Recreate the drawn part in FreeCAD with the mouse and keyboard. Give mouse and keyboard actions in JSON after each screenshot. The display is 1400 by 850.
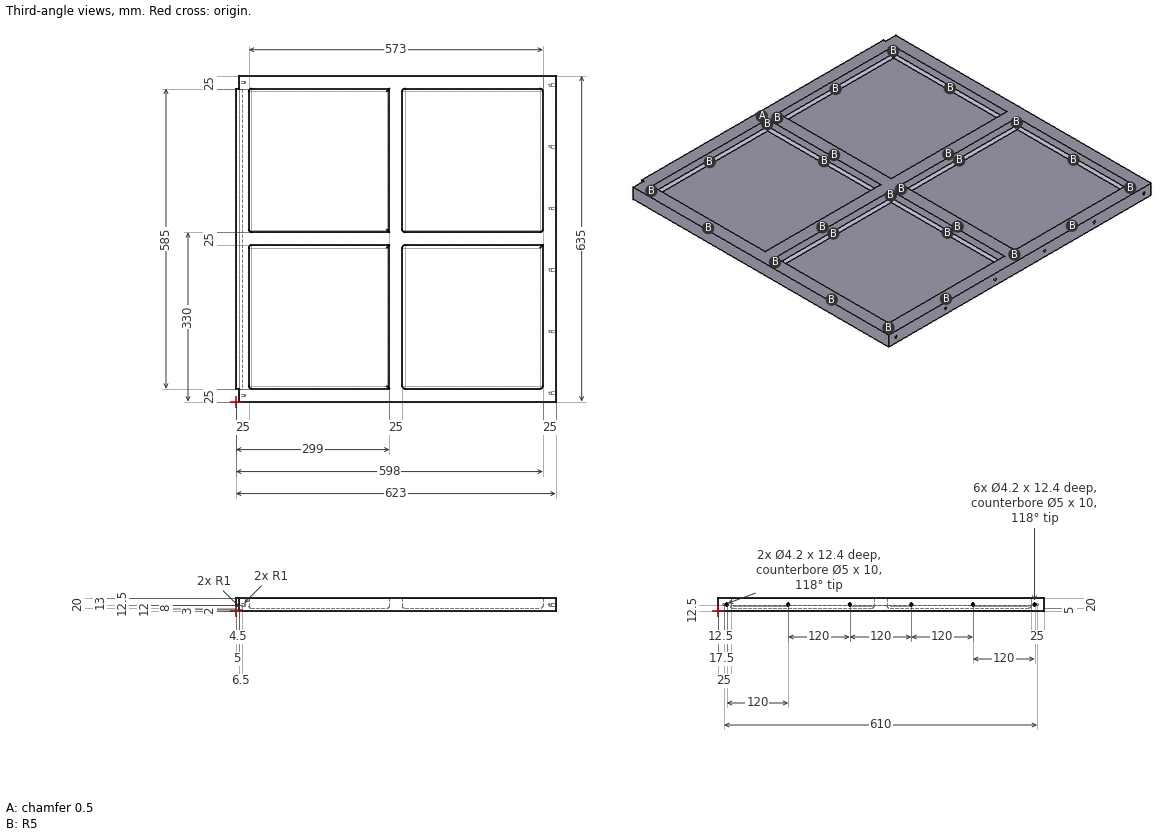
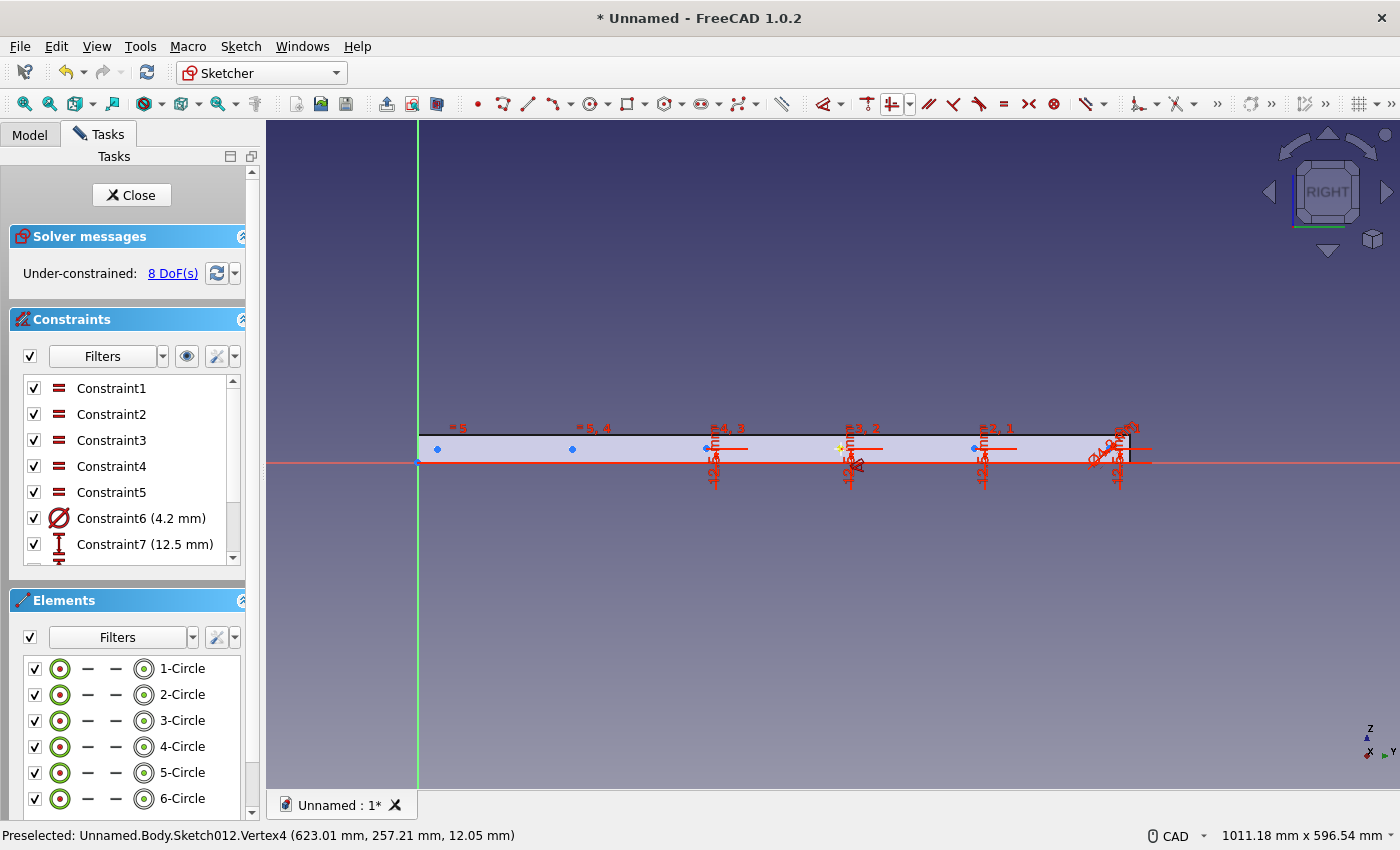
{"action": "scroll", "coordinate": [572, 449], "scroll_direction": "up", "scroll_amount": 6}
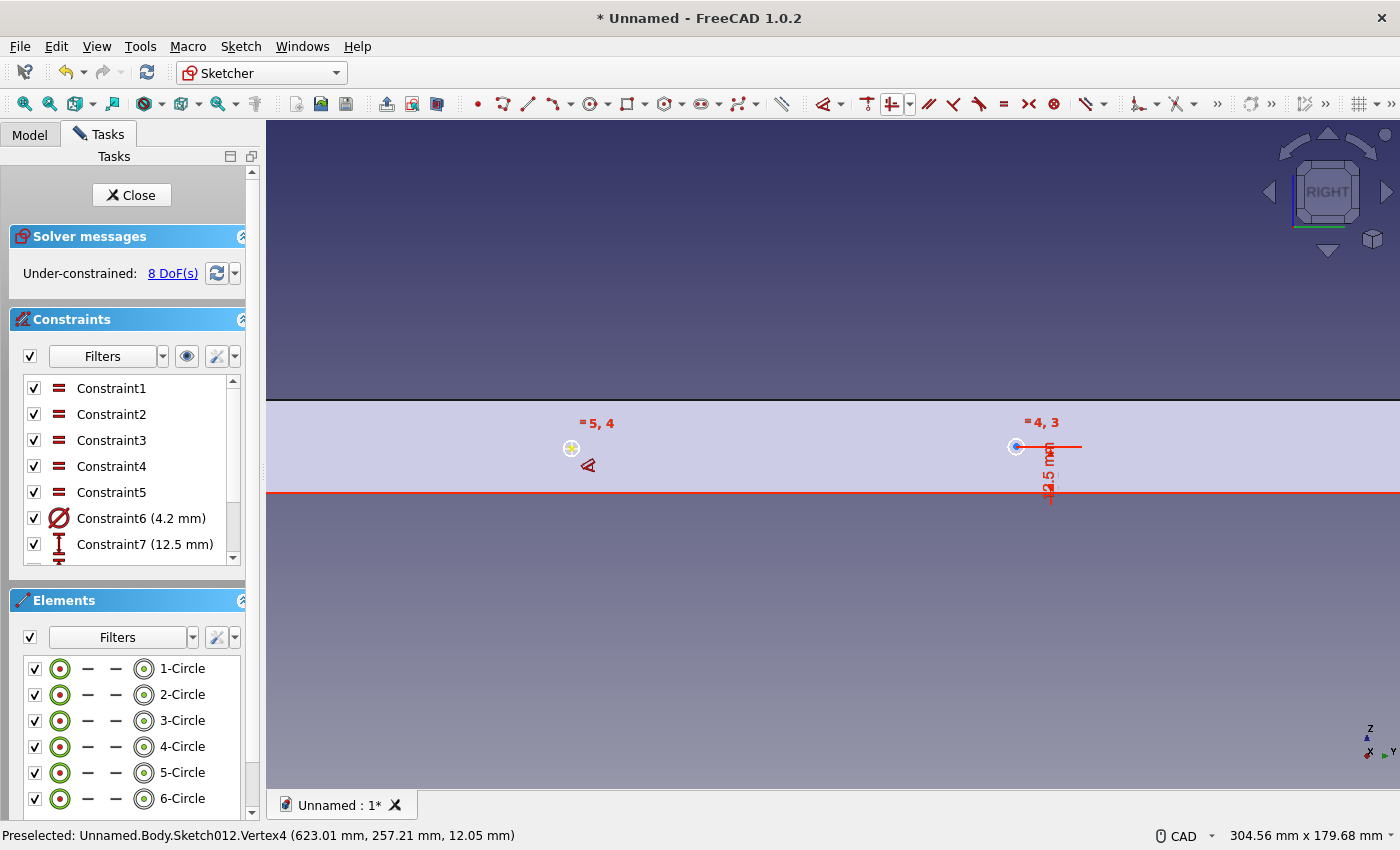
{"action": "left_click", "coordinate": [571, 448]}
{"action": "left_click", "coordinate": [605, 471]}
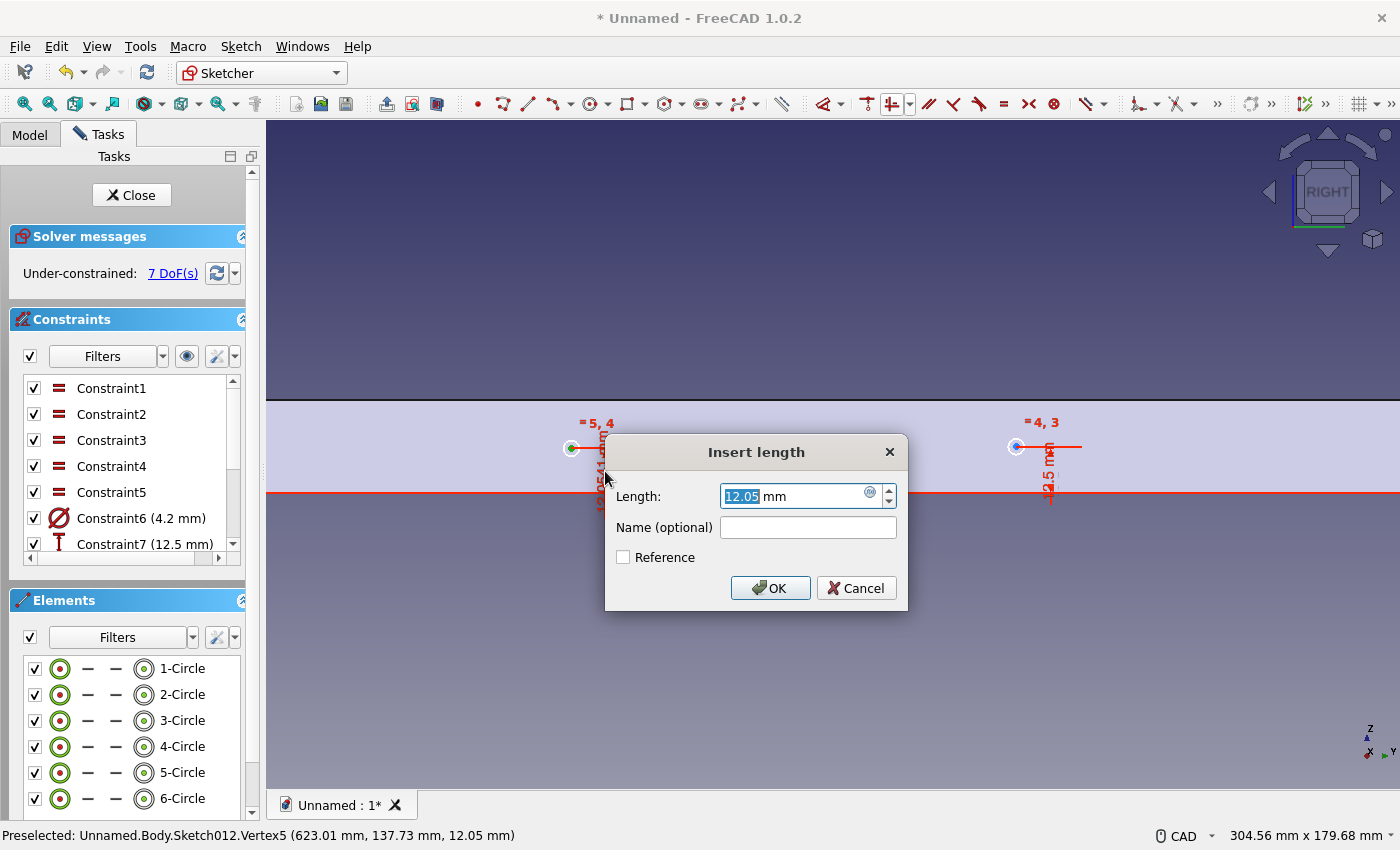
{"action": "type", "text": "12.5"}
{"action": "key", "text": "Return"}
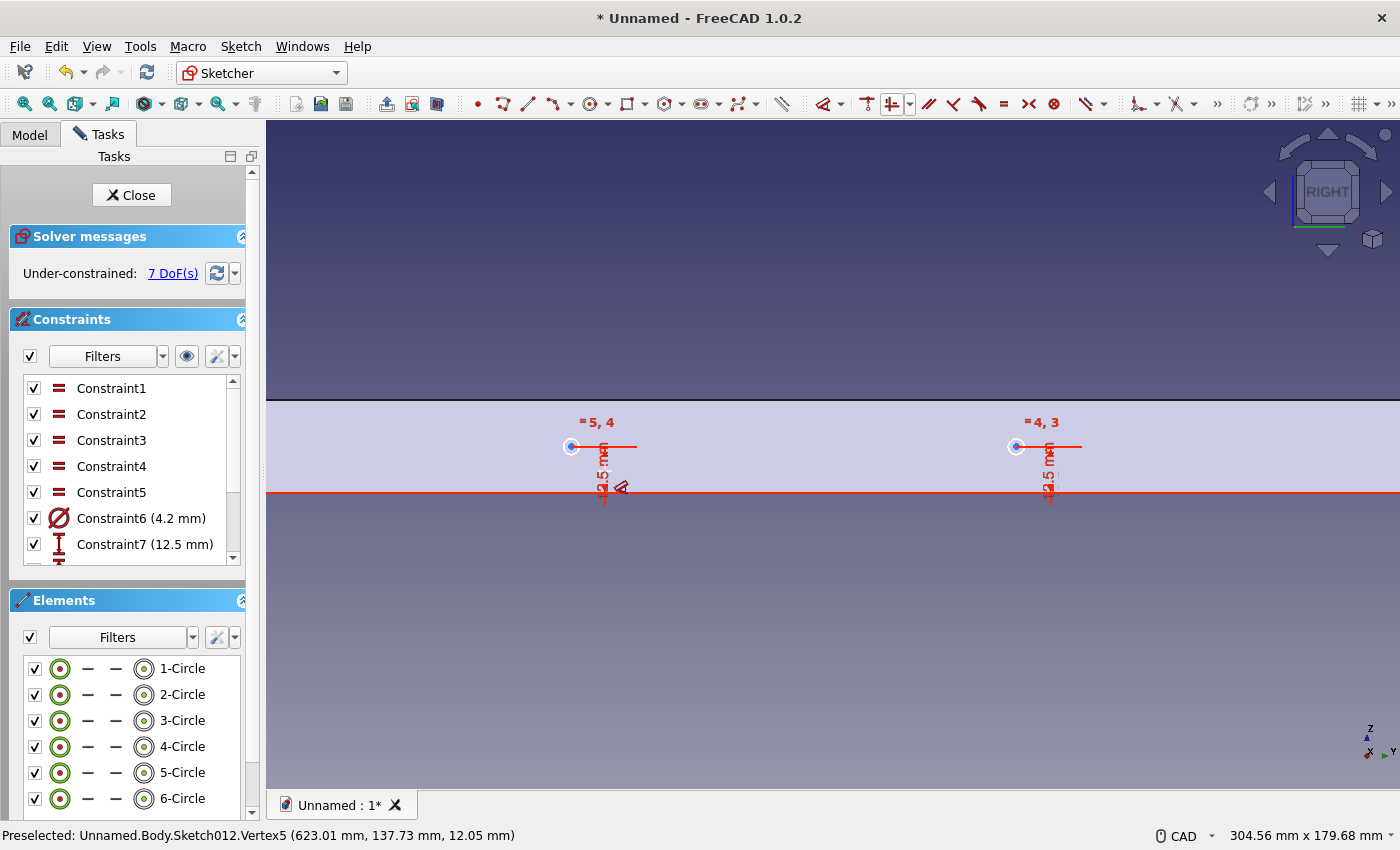
{"action": "scroll", "coordinate": [572, 449], "scroll_direction": "down", "scroll_amount": 6}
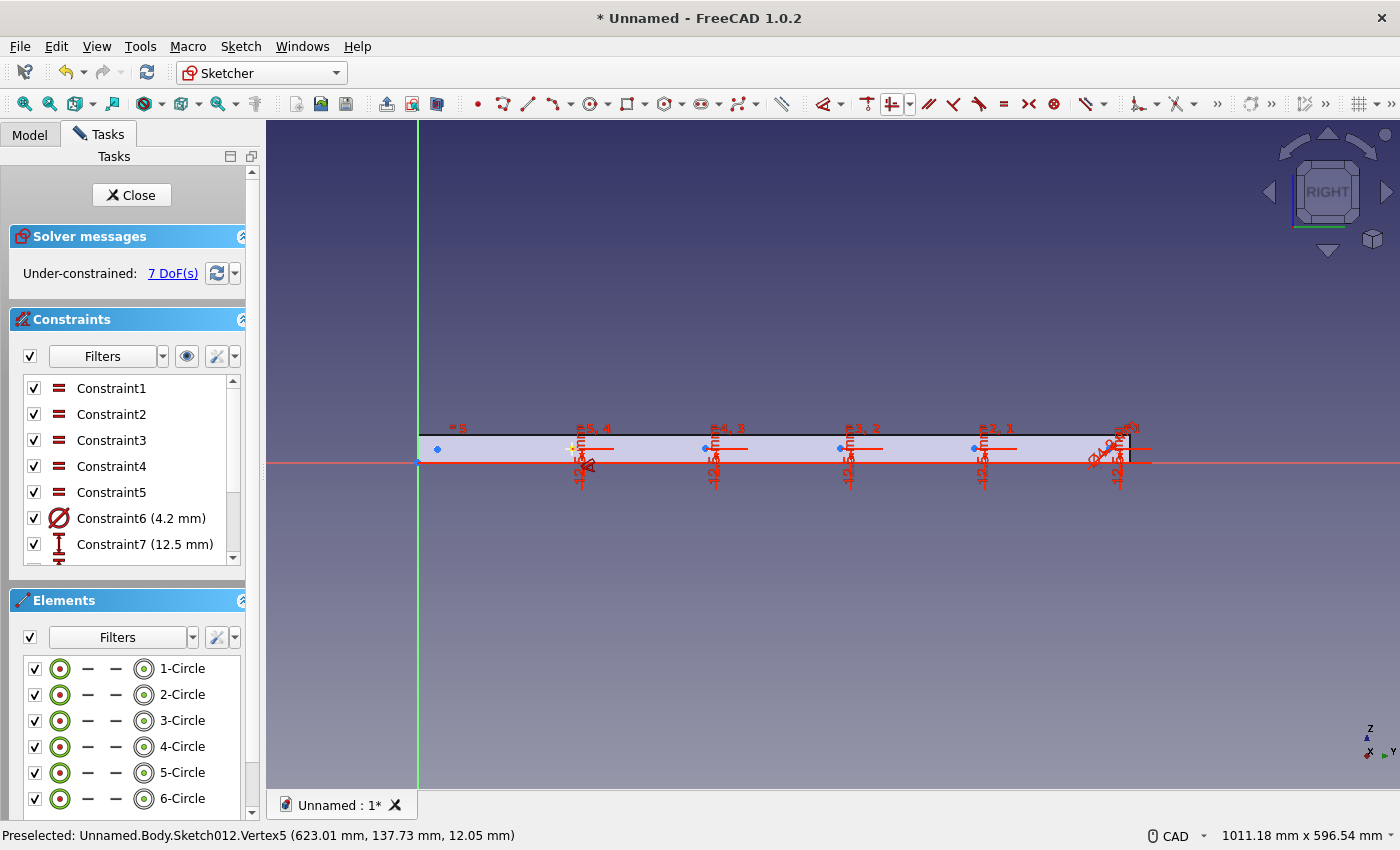
{"action": "scroll", "coordinate": [437, 449], "scroll_direction": "up", "scroll_amount": 4}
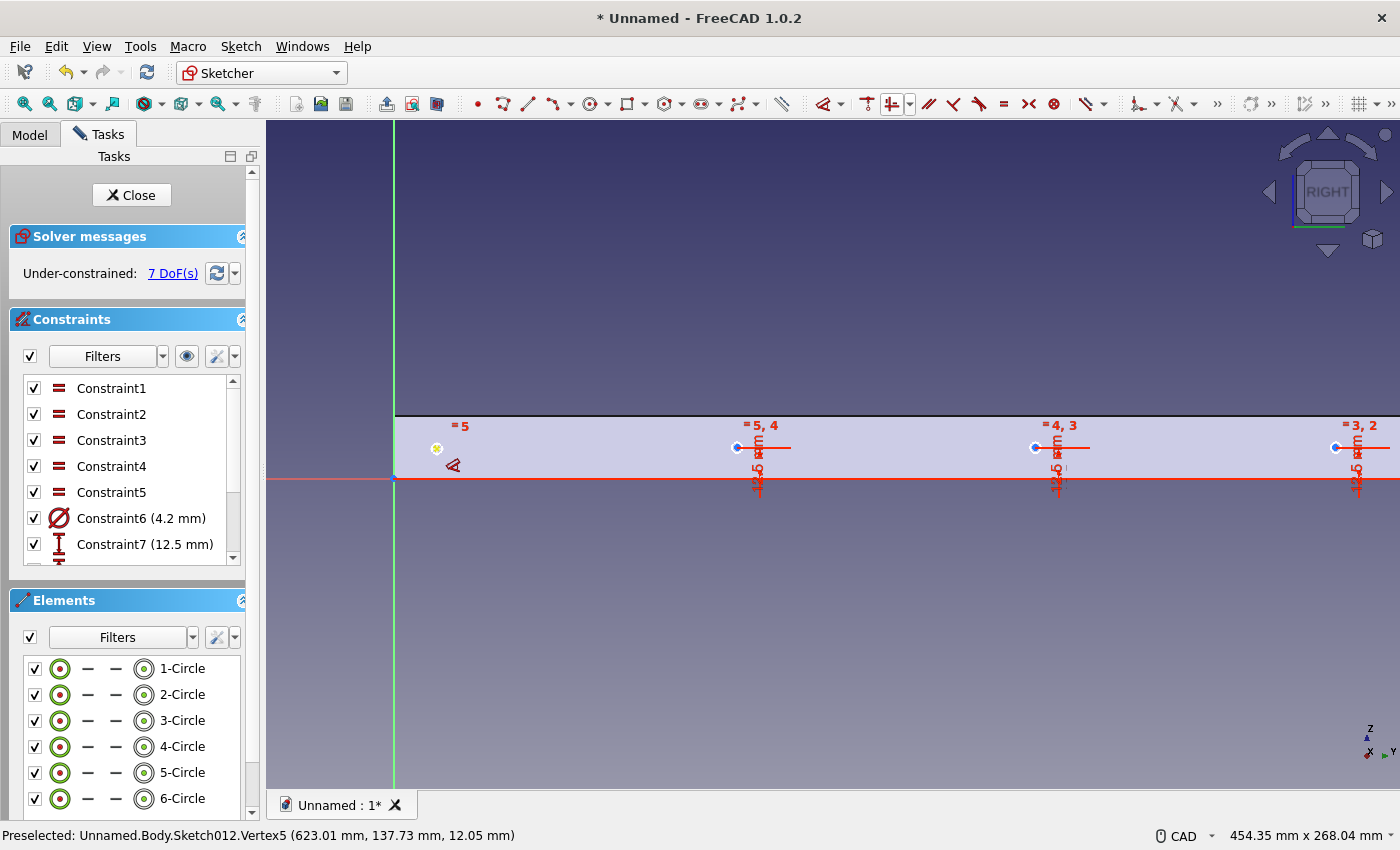
{"action": "left_click", "coordinate": [437, 449]}
{"action": "left_click", "coordinate": [415, 513]}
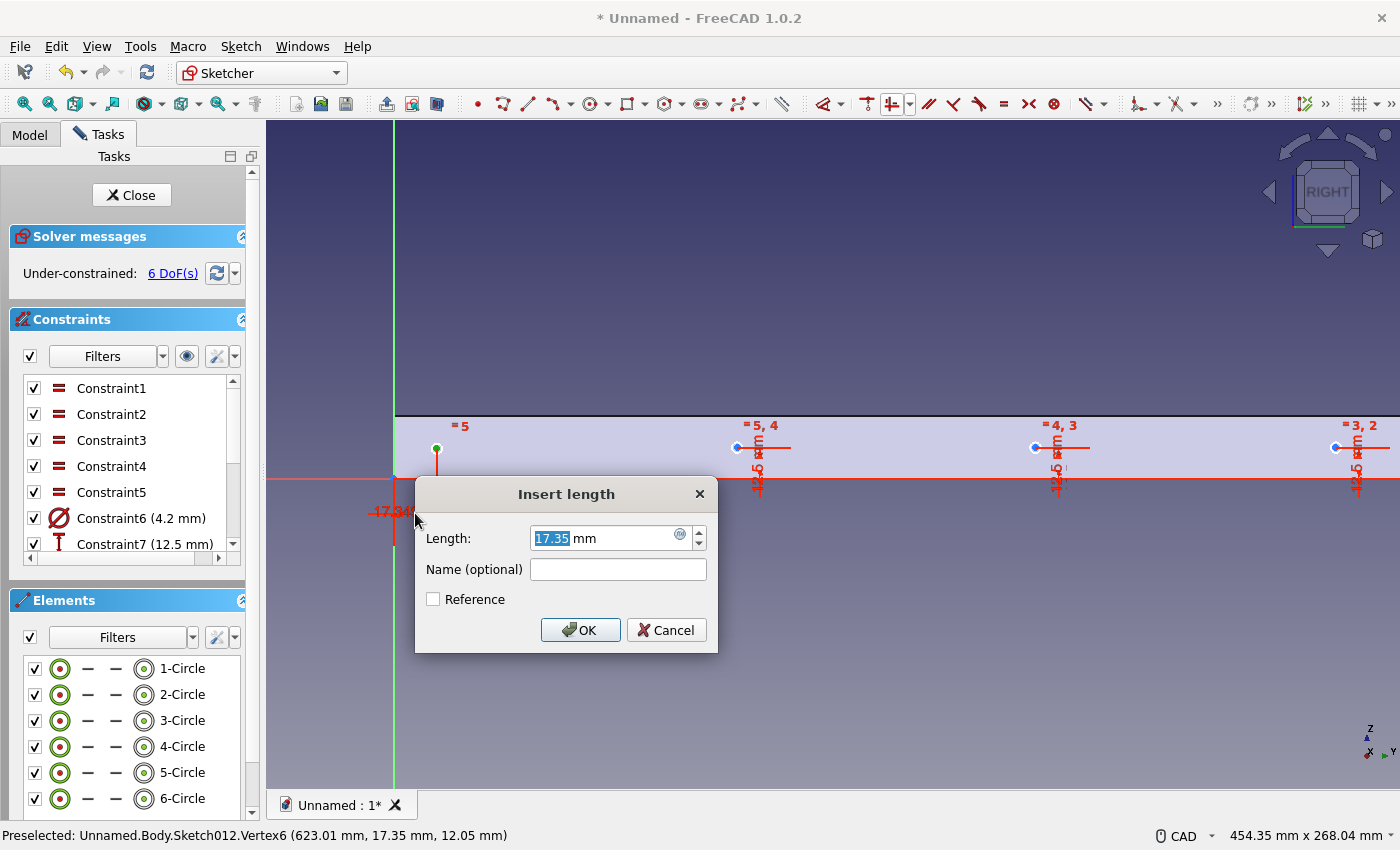
{"action": "type", "text": "17.5"}
{"action": "key", "text": "Return"}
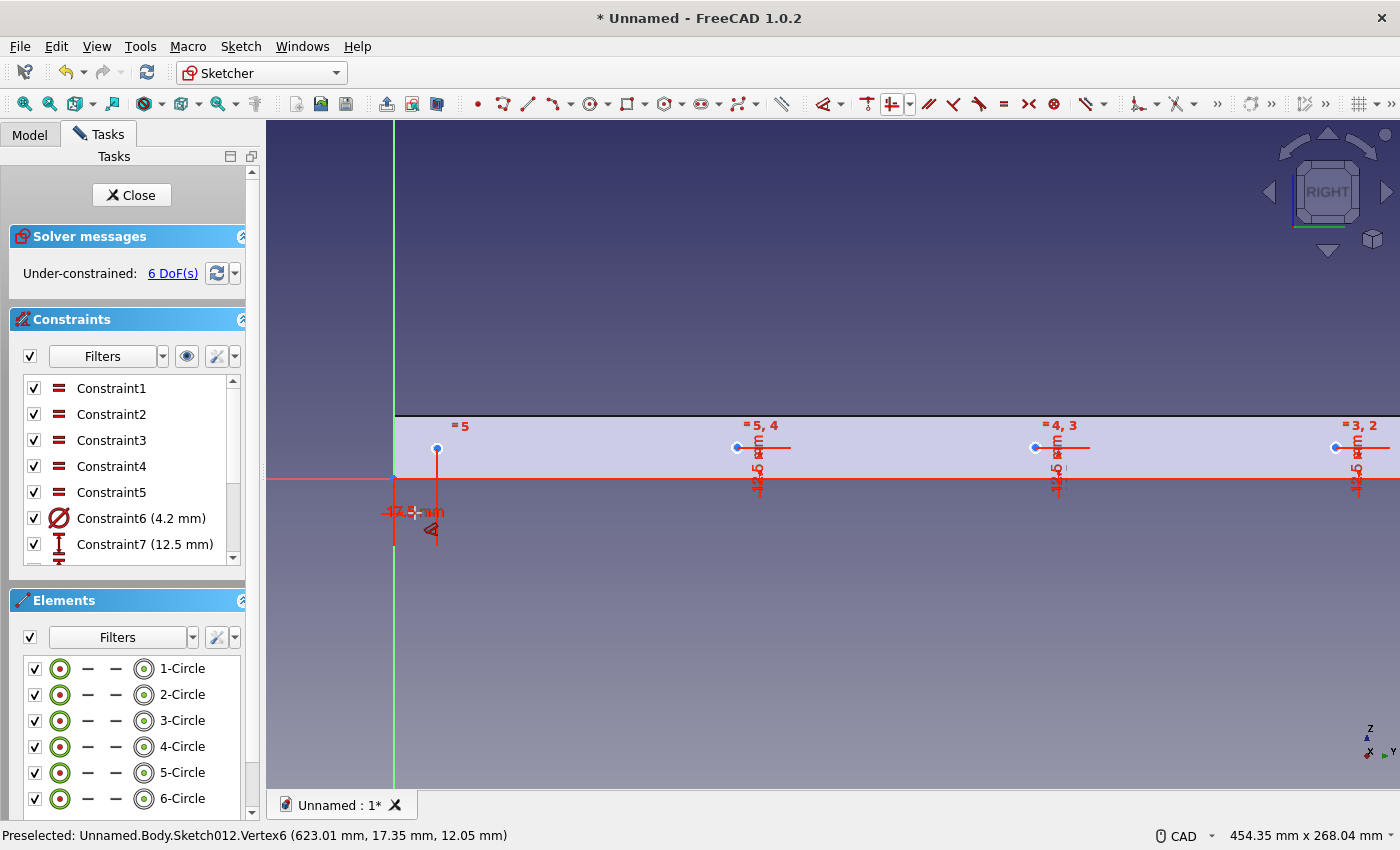
{"action": "scroll", "coordinate": [437, 449], "scroll_direction": "up", "scroll_amount": 2}